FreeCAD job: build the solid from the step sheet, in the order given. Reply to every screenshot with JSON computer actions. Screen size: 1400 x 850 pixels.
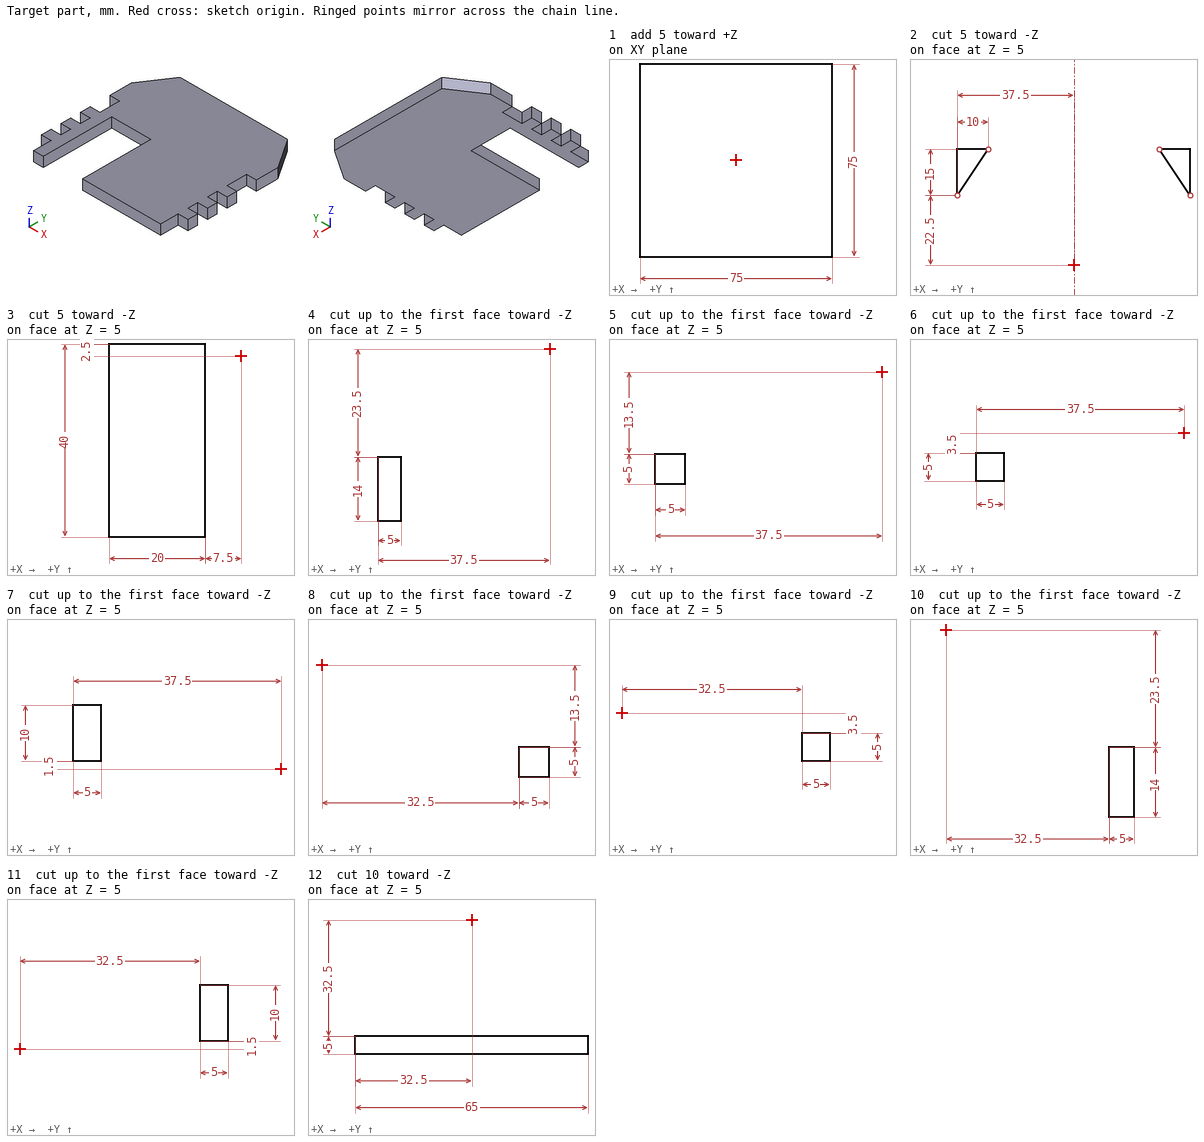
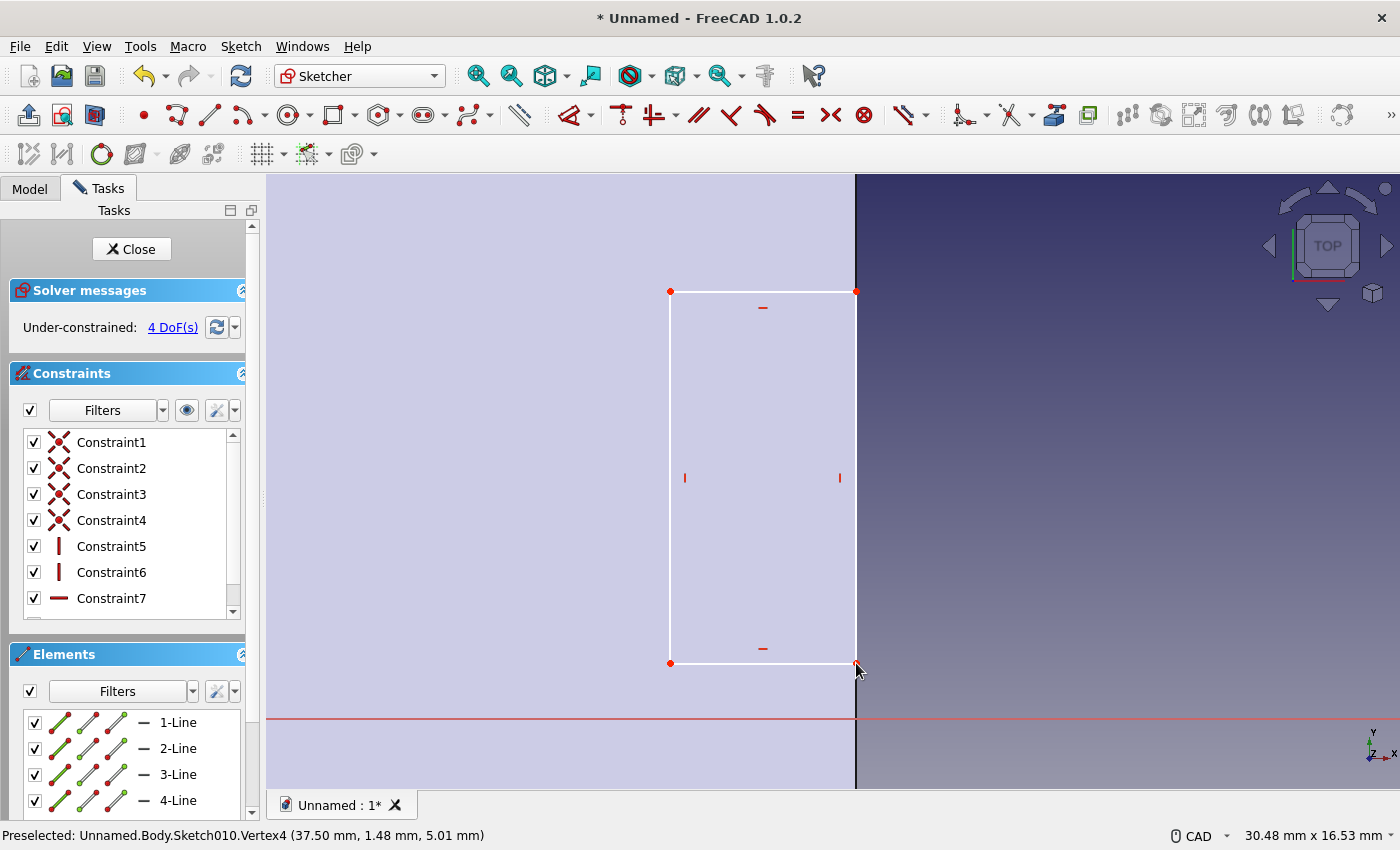
{"action": "left_click", "coordinate": [568, 116]}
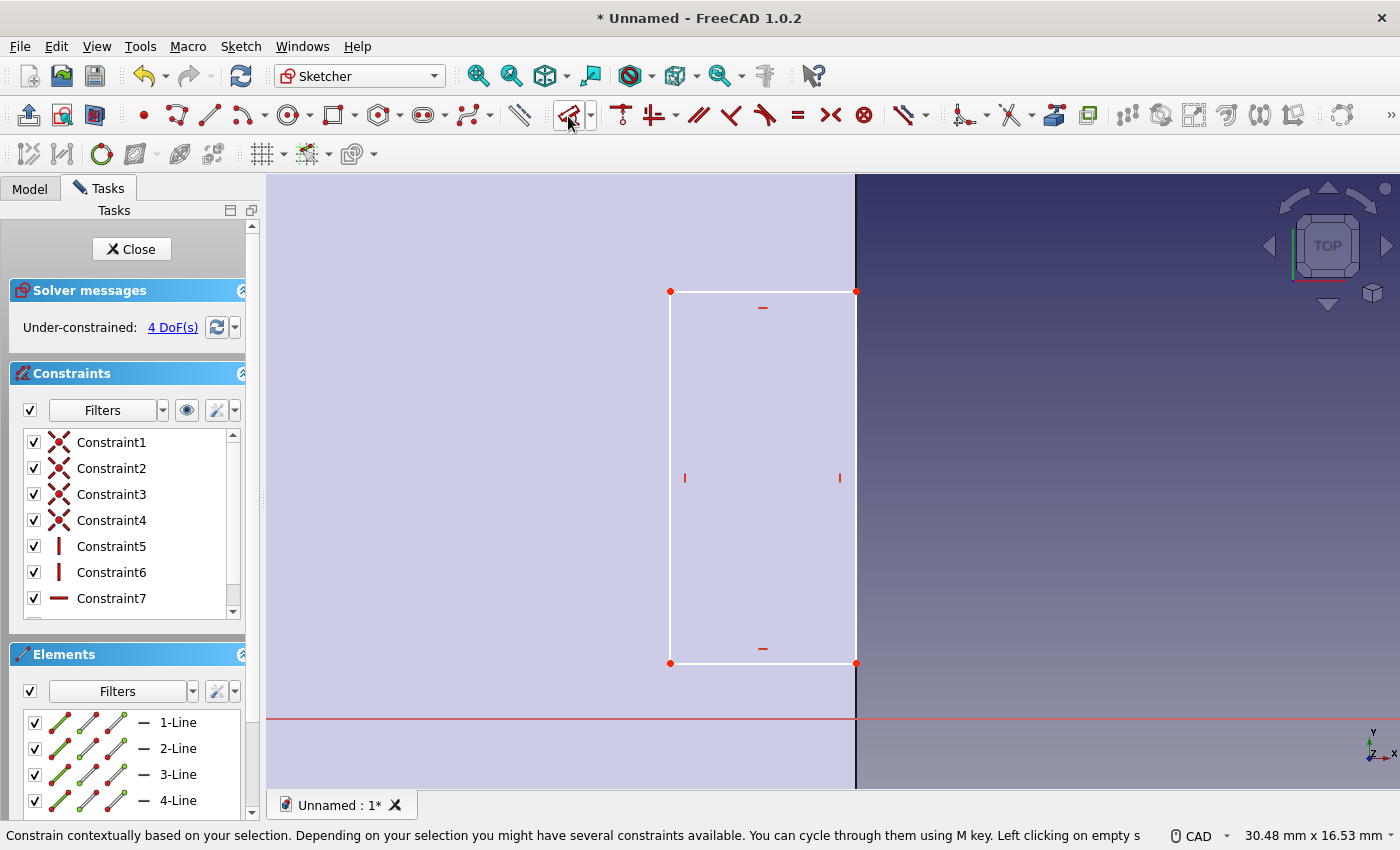
{"action": "left_click", "coordinate": [726, 664]}
{"action": "left_click", "coordinate": [763, 698]}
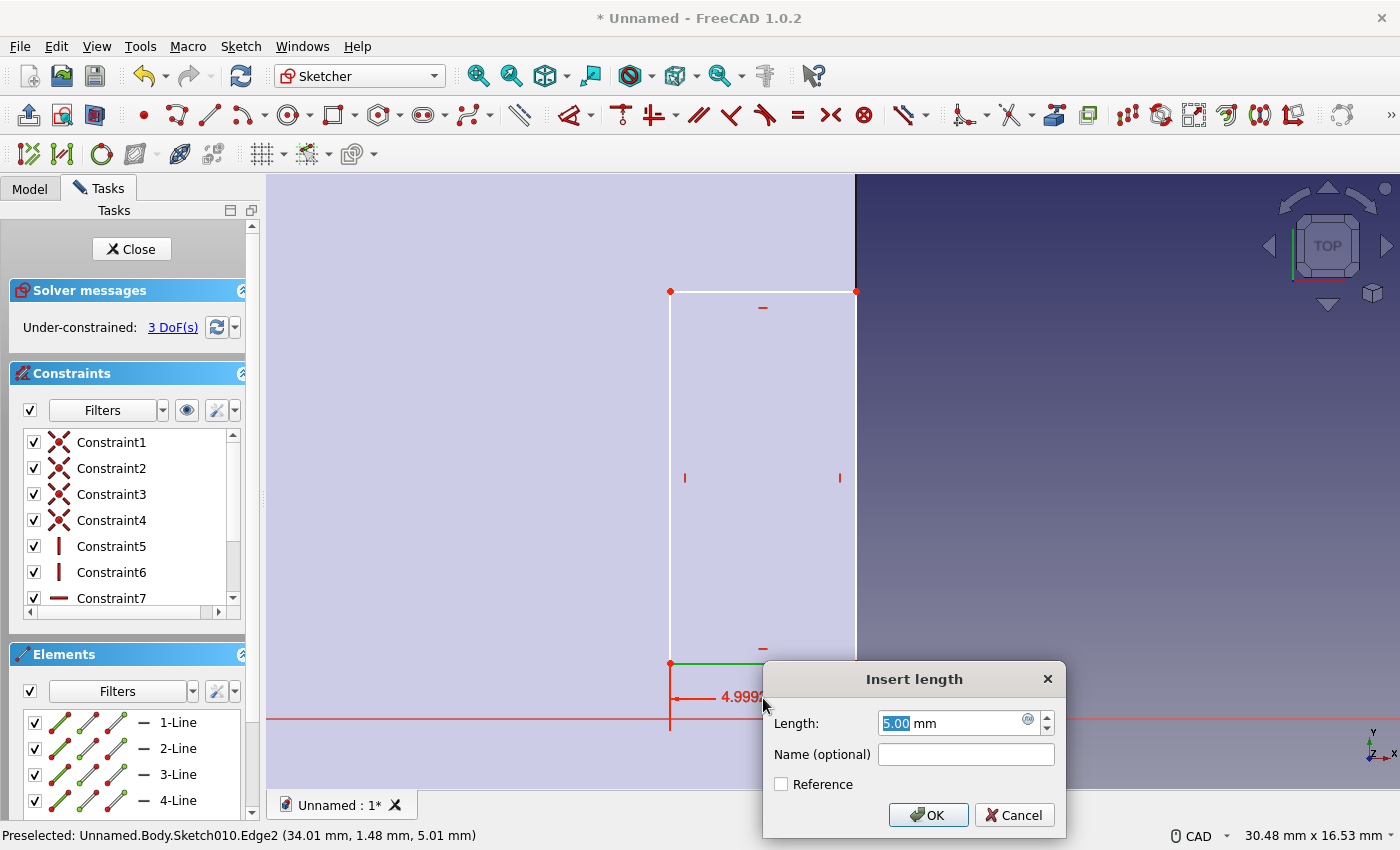
{"action": "type", "text": "5"}
{"action": "key", "text": "Return"}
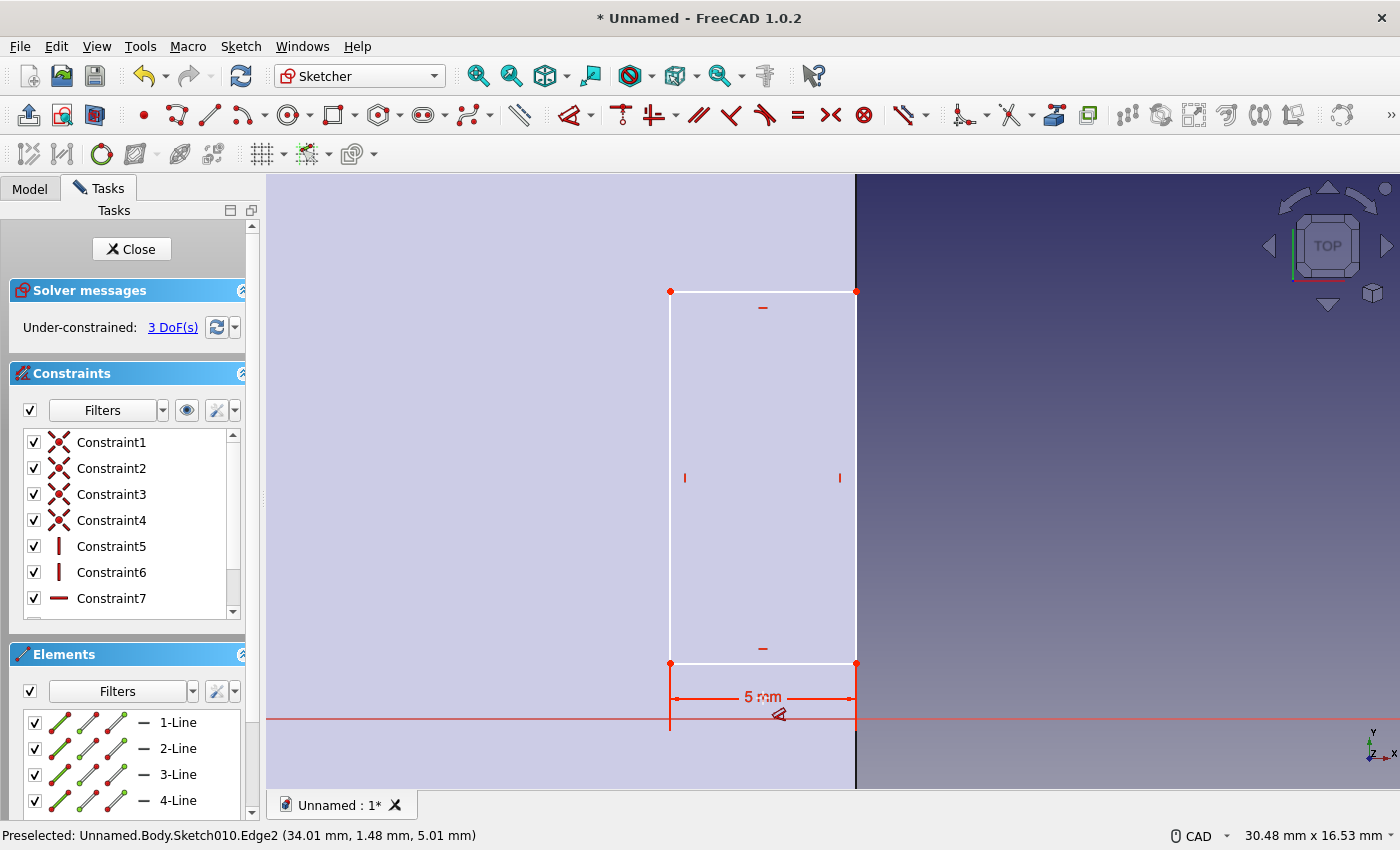
{"action": "left_click", "coordinate": [670, 404]}
{"action": "left_click", "coordinate": [636, 478]}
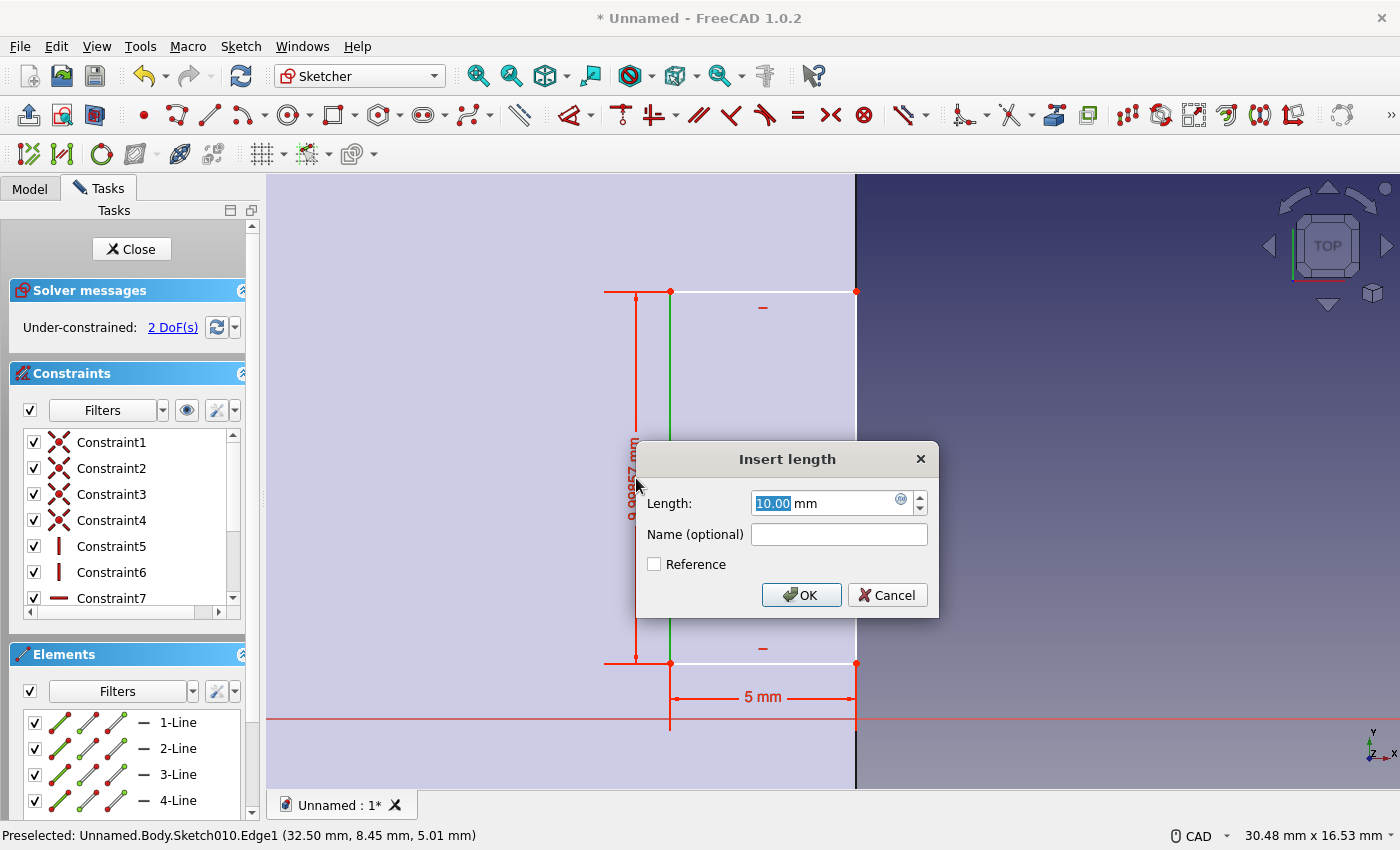
{"action": "type", "text": "10"}
{"action": "key", "text": "Return"}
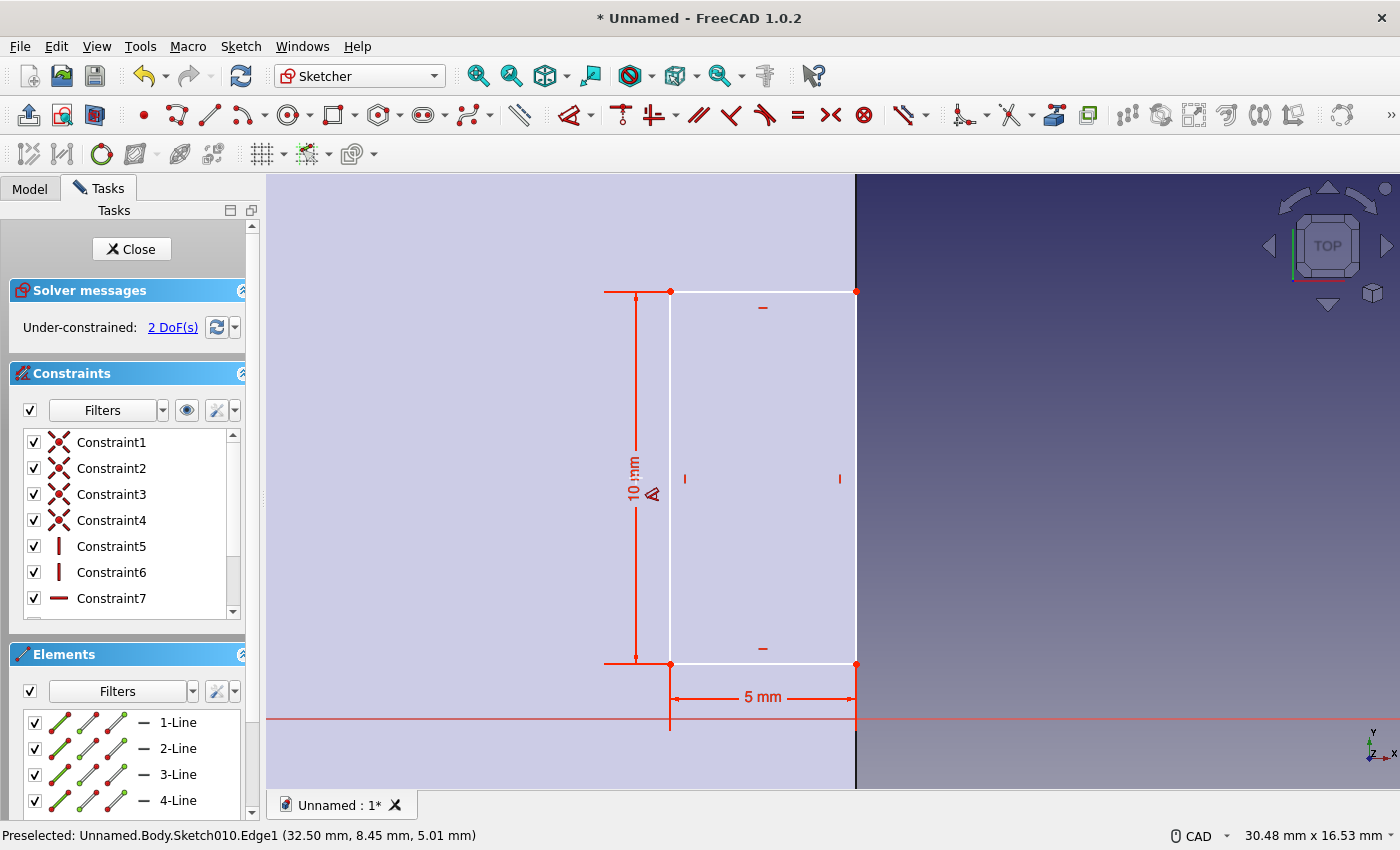
{"action": "left_click", "coordinate": [670, 664]}
{"action": "left_click", "coordinate": [850, 692]}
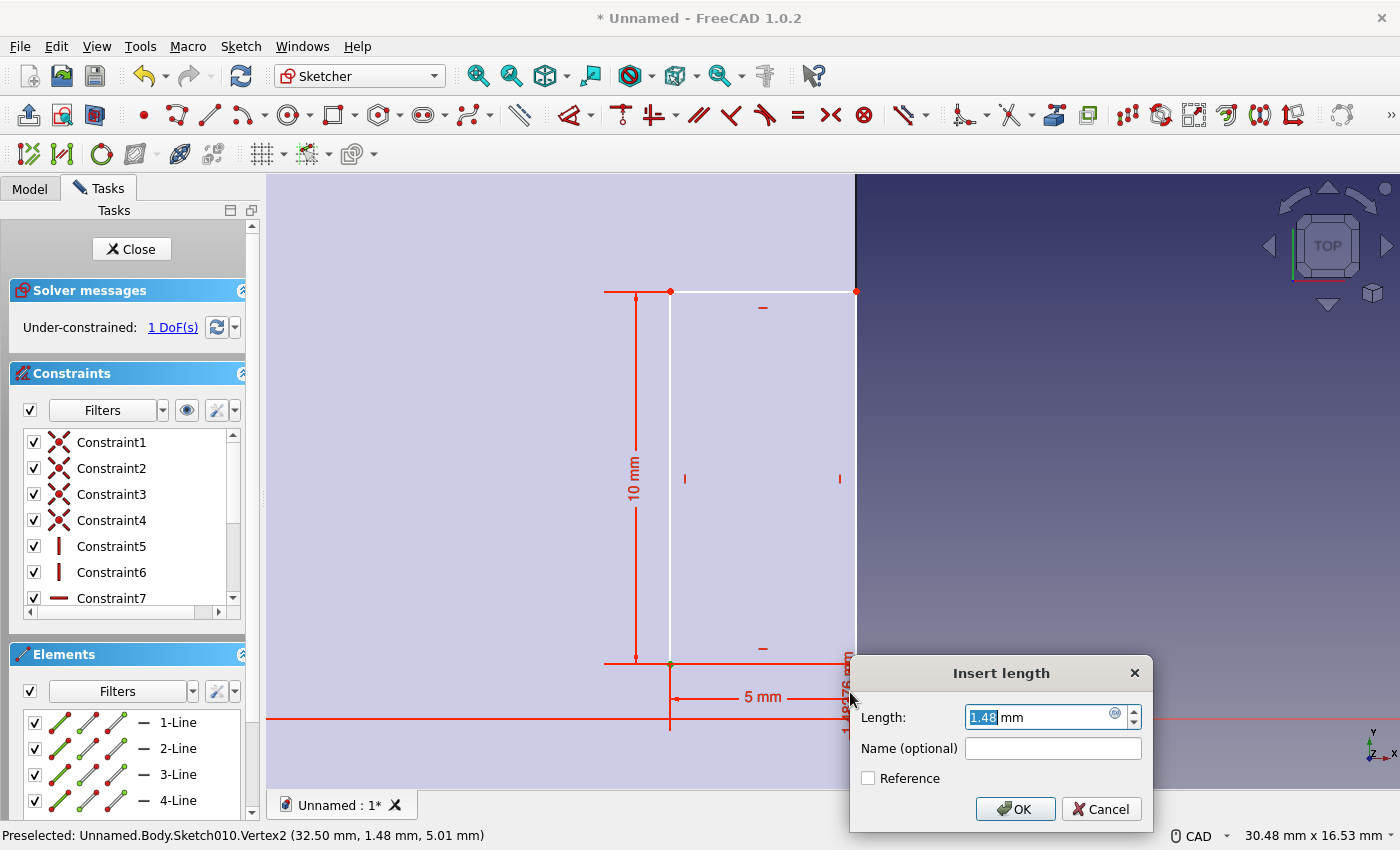
{"action": "type", "text": "1.5"}
{"action": "key", "text": "Return"}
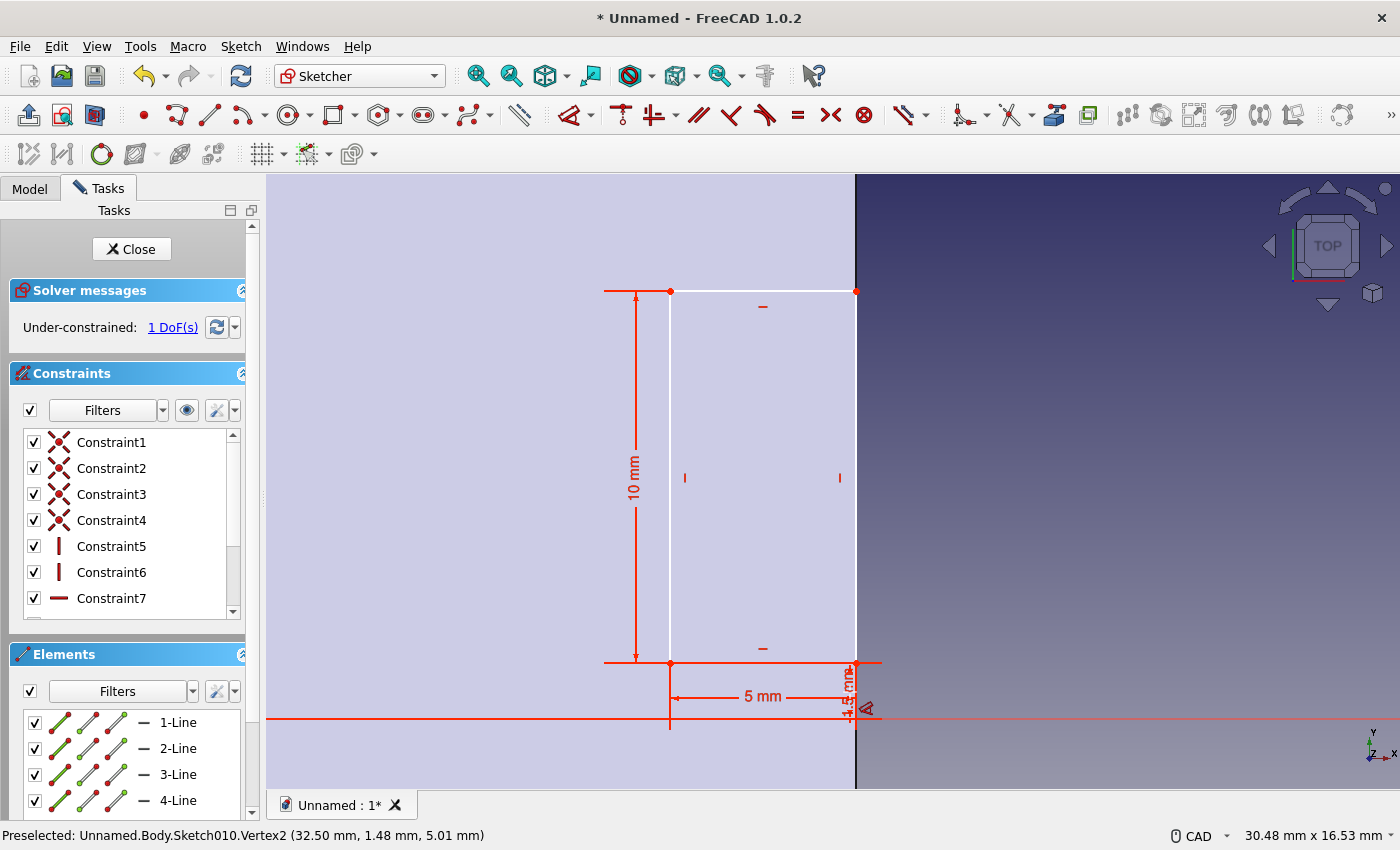
{"action": "left_click", "coordinate": [670, 291]}
{"action": "left_click", "coordinate": [482, 753]}